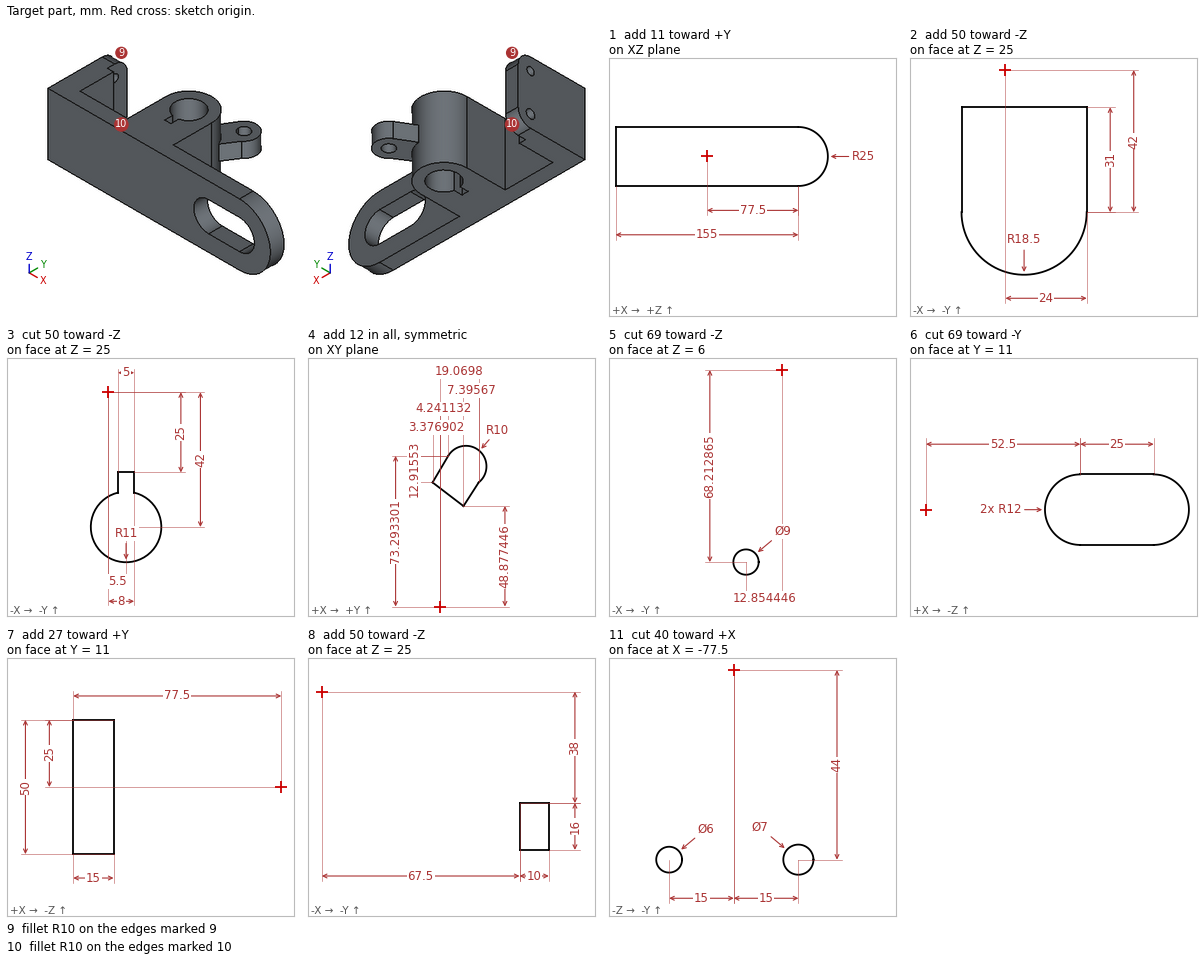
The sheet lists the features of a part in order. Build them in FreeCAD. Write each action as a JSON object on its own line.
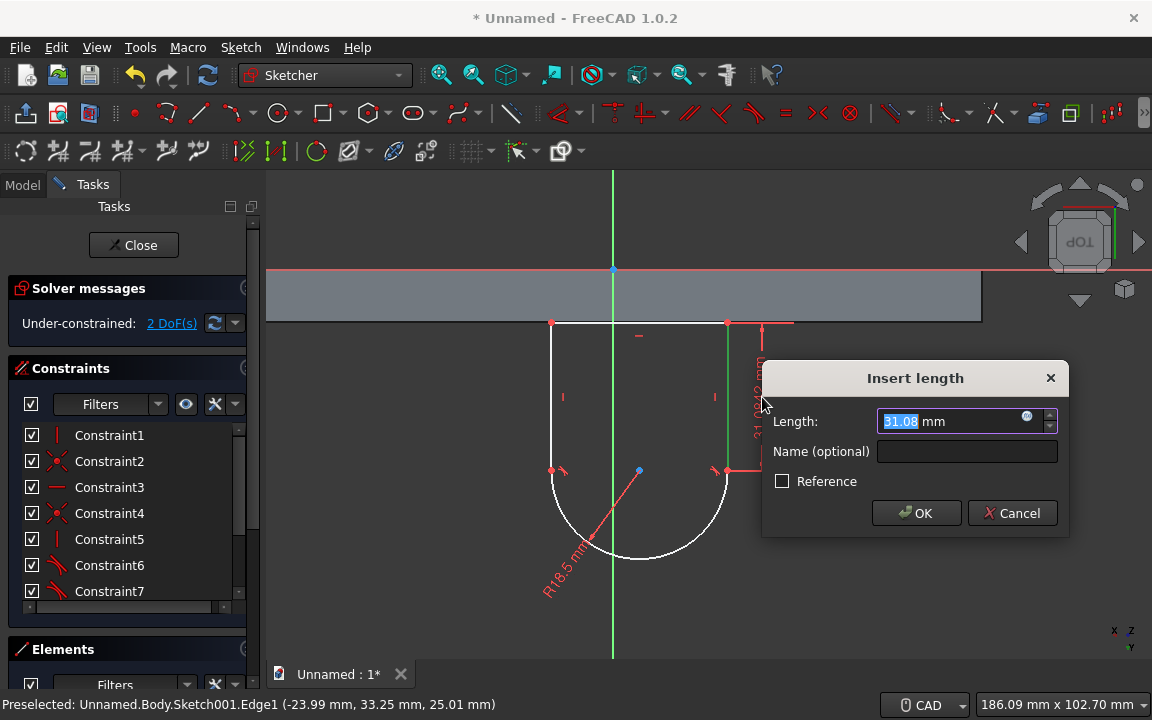
{"action": "type", "text": "31"}
{"action": "key", "text": "Return"}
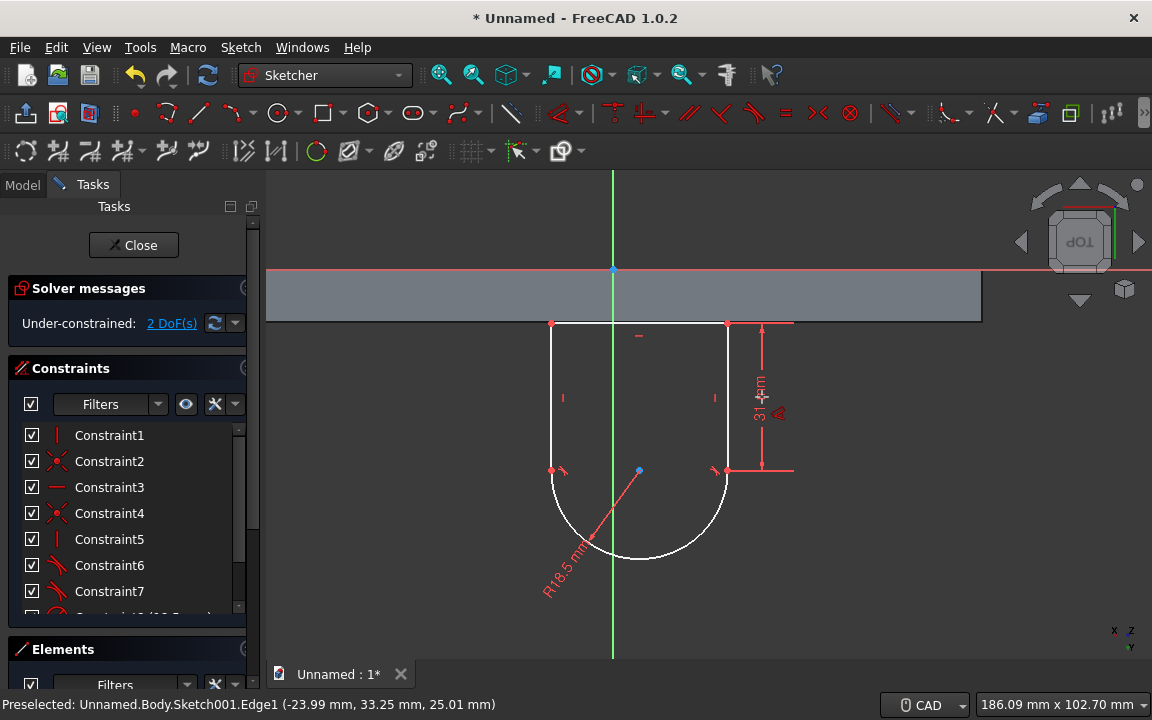
{"action": "left_click", "coordinate": [728, 471]}
{"action": "left_click", "coordinate": [670, 236]}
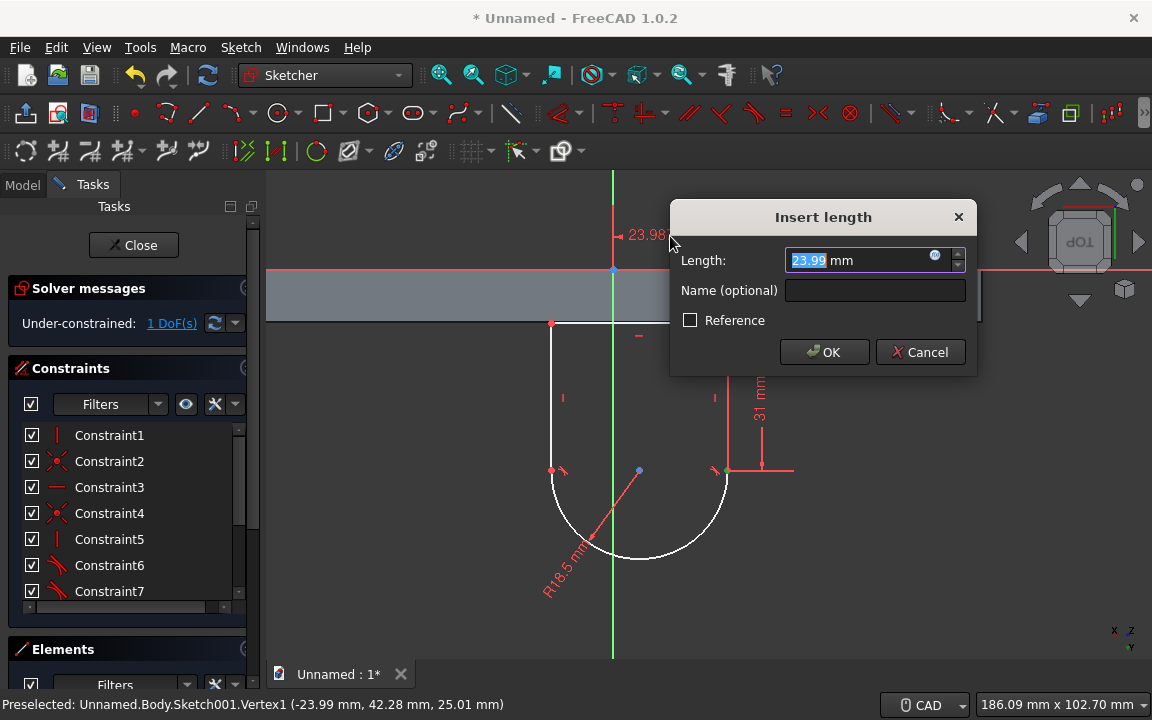
{"action": "type", "text": "24"}
{"action": "key", "text": "Return"}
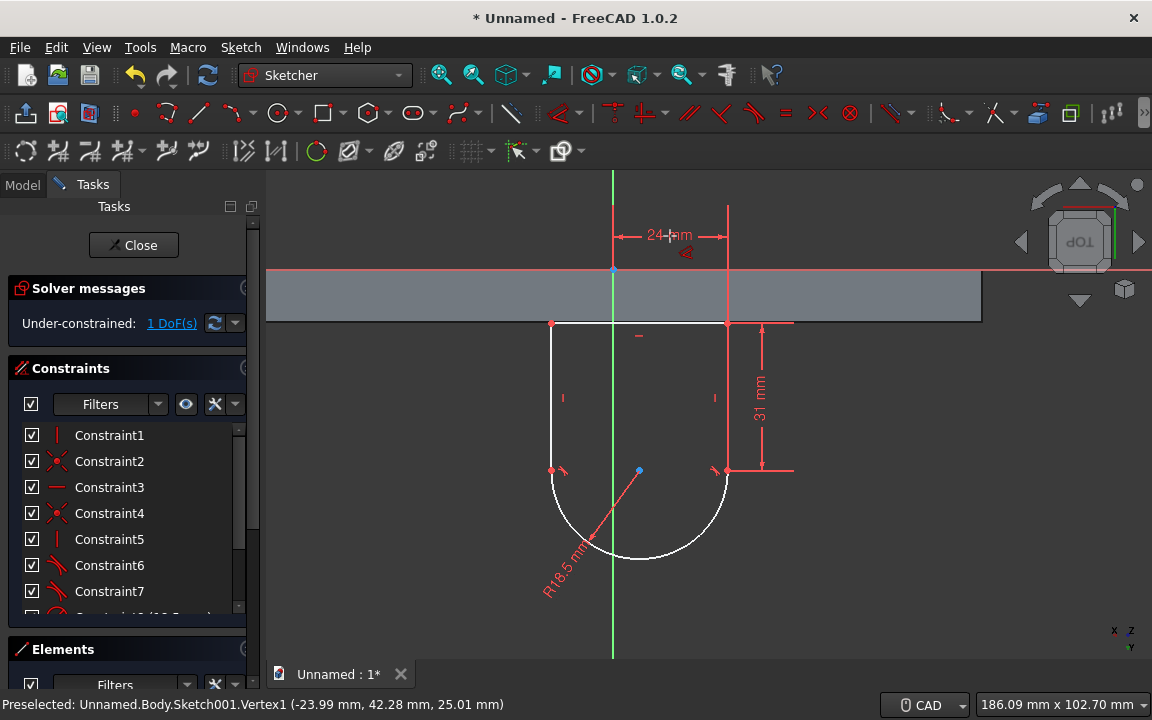
{"action": "left_click", "coordinate": [728, 471]}
{"action": "left_click", "coordinate": [762, 370]}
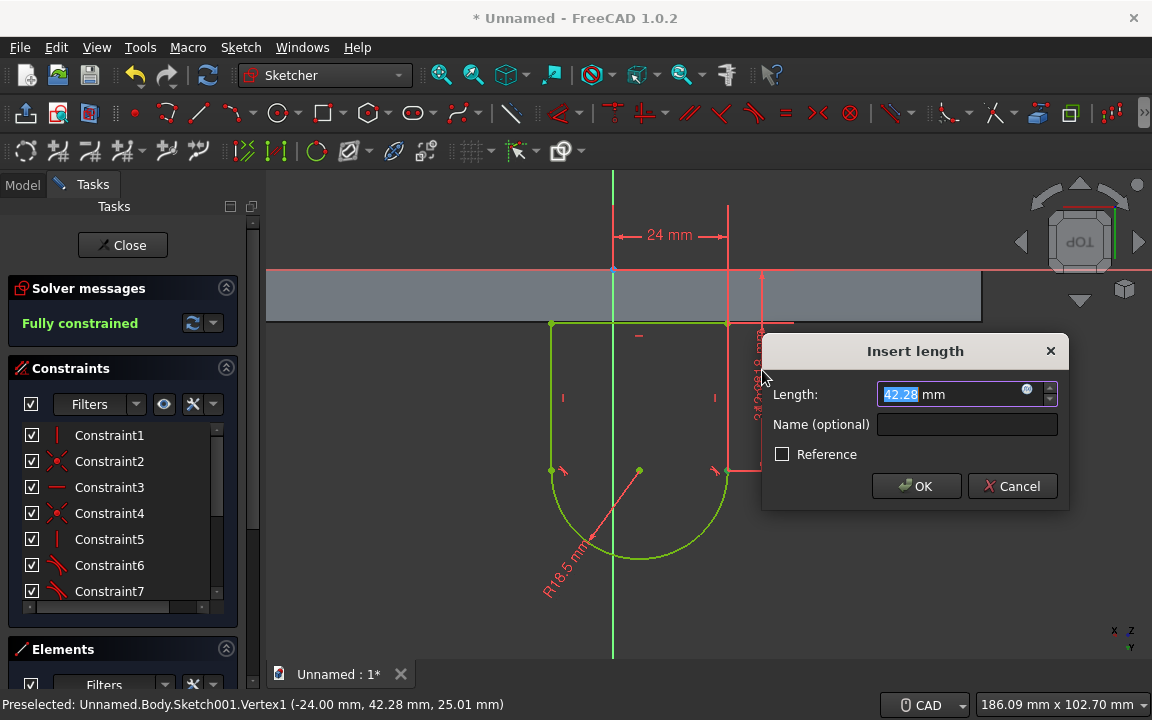
{"action": "type", "text": "42"}
{"action": "key", "text": "Return"}
{"action": "key", "text": "Escape"}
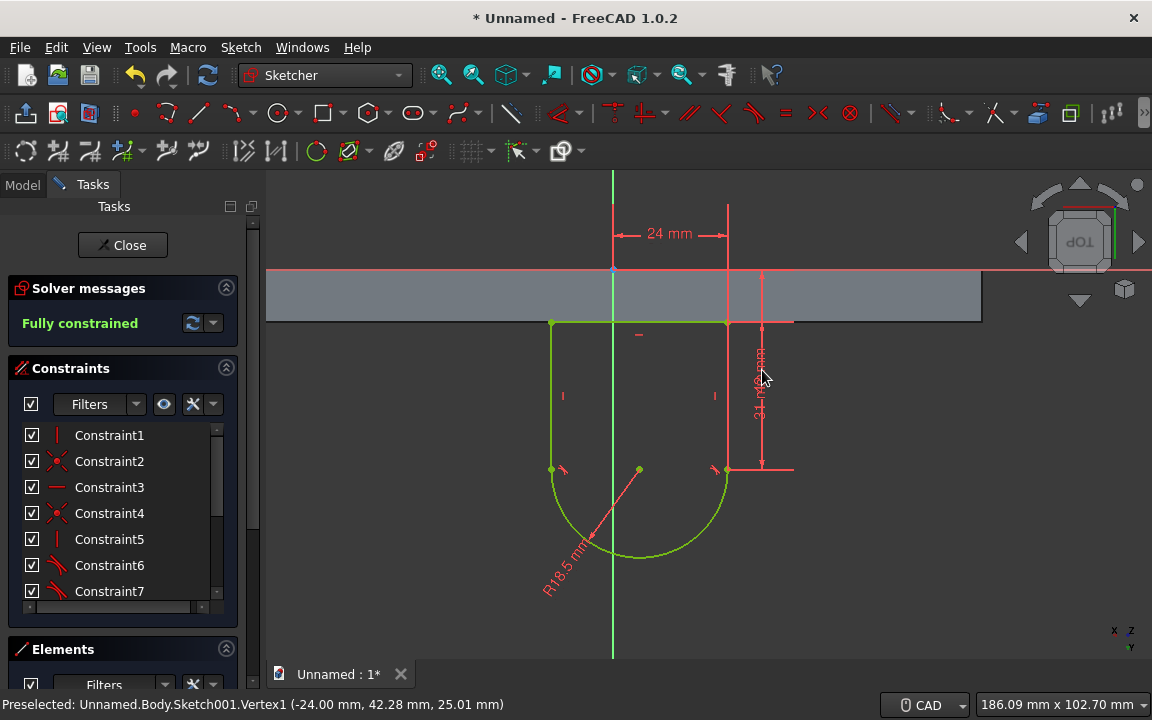
{"action": "left_click", "coordinate": [123, 245]}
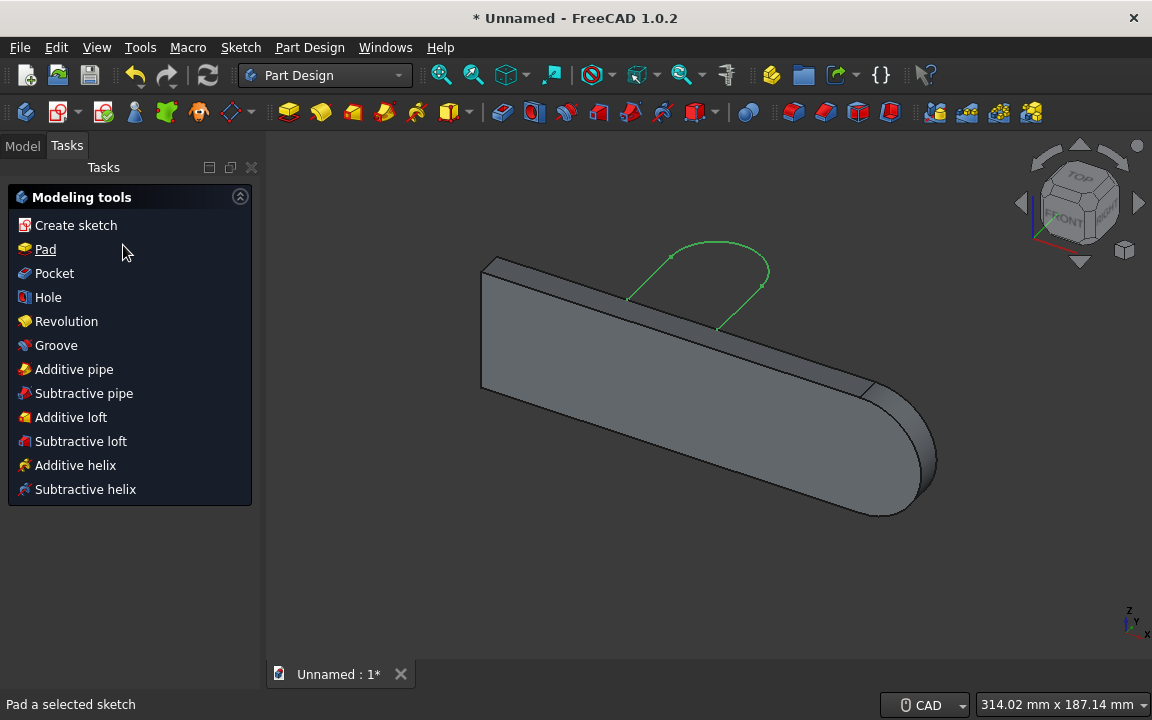
{"action": "left_click", "coordinate": [290, 112]}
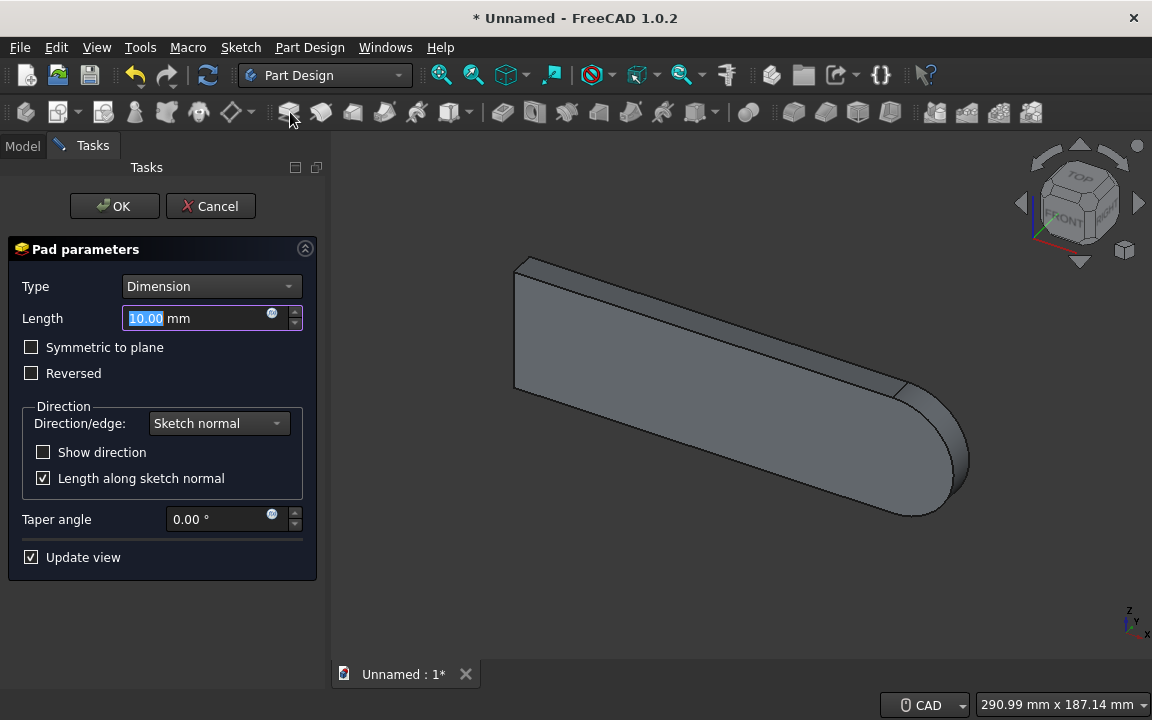
{"action": "type", "text": "50"}
{"action": "key", "text": "Tab"}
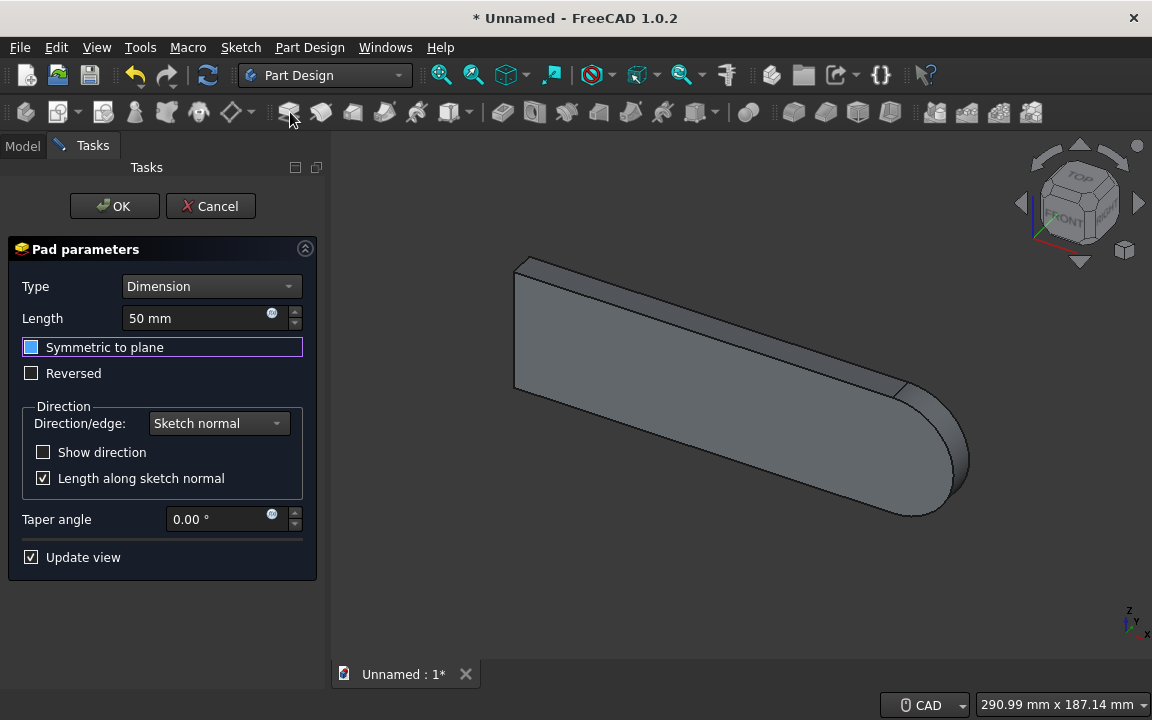
{"action": "left_click", "coordinate": [30, 373]}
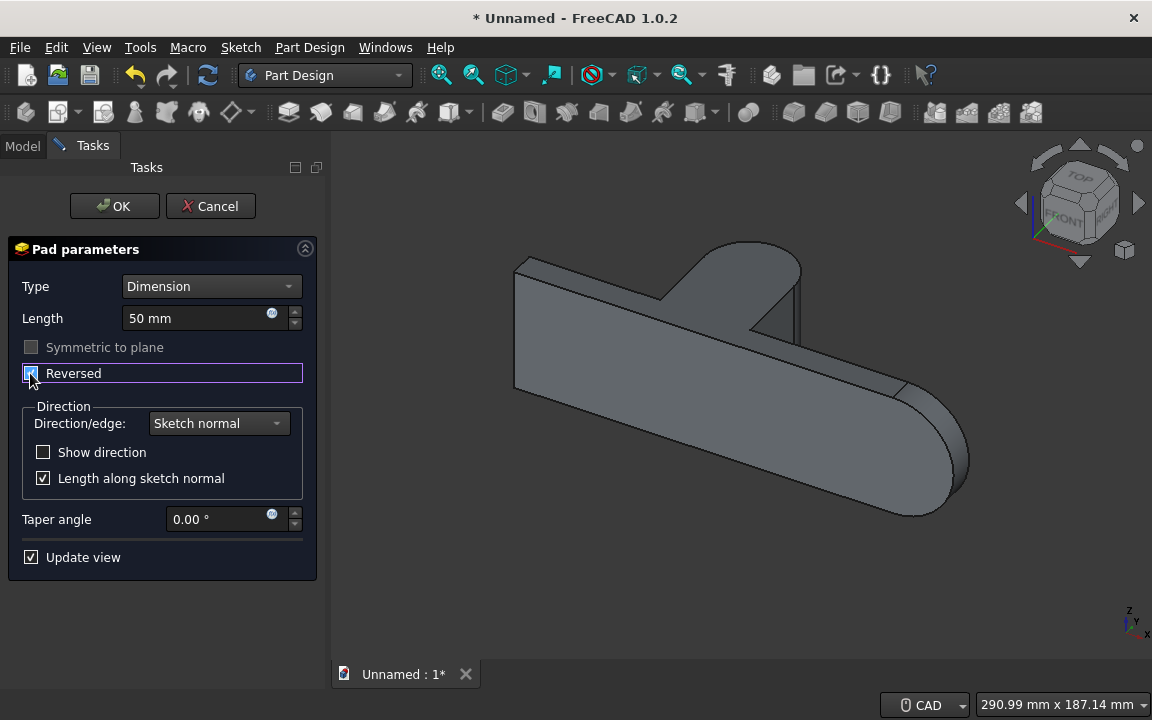
{"action": "left_click", "coordinate": [115, 206]}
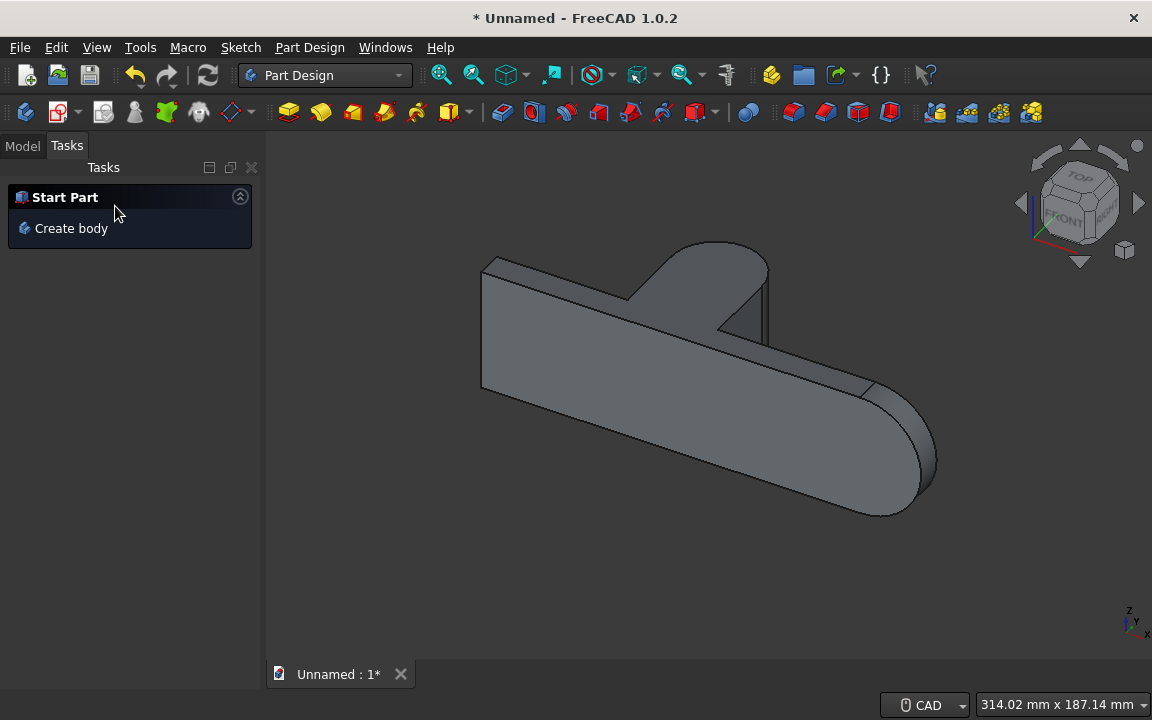
{"action": "left_click", "coordinate": [726, 279]}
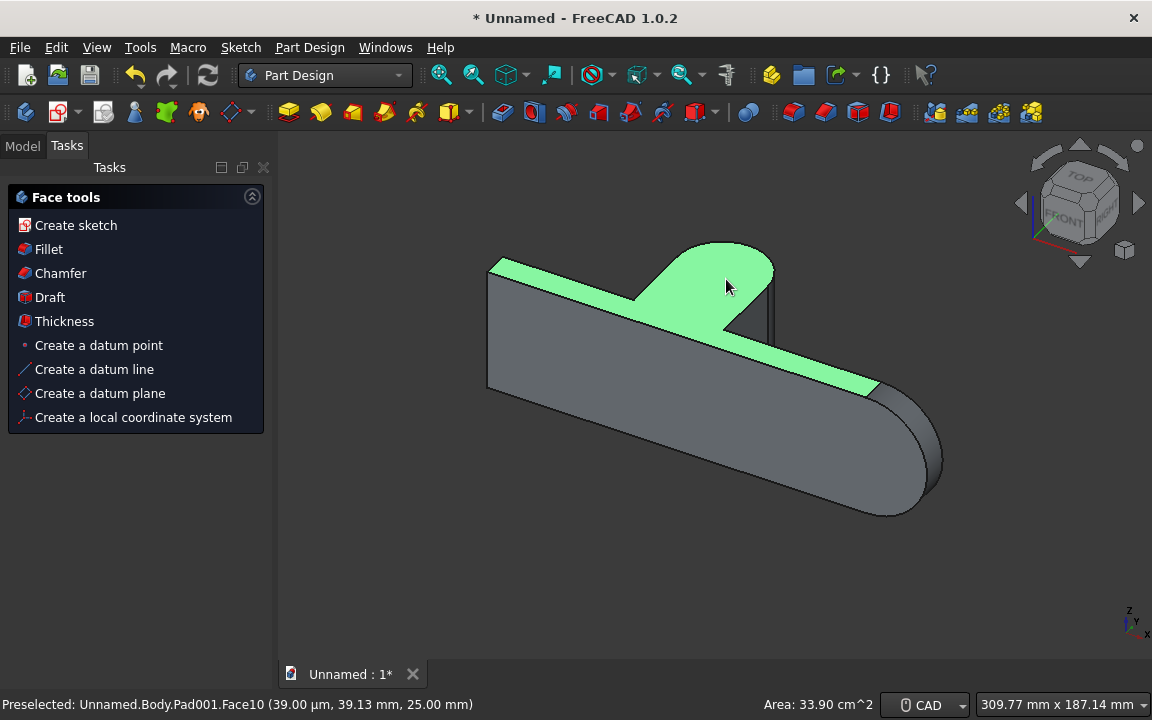
{"action": "left_click", "coordinate": [58, 112]}